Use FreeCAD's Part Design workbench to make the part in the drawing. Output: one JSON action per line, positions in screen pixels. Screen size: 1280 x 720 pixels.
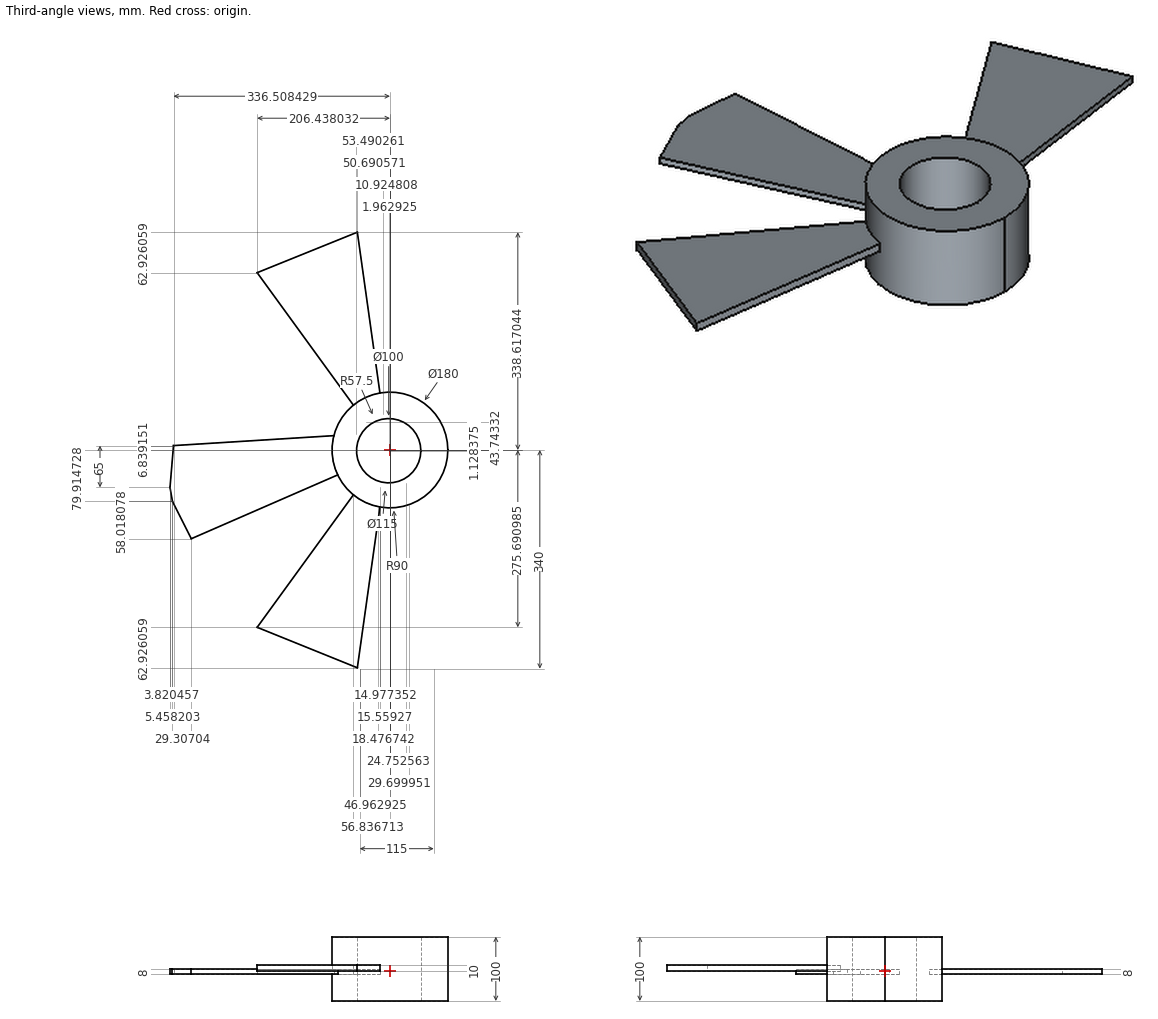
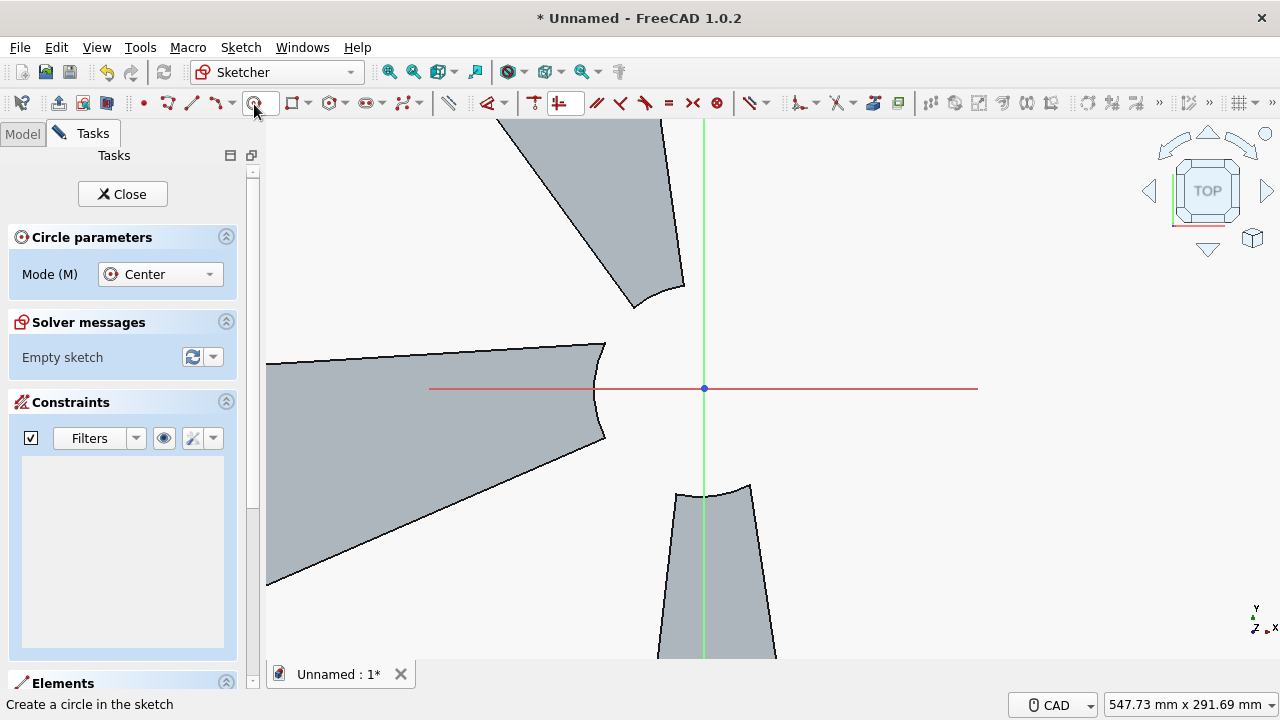
{"action": "left_click", "coordinate": [704, 389]}
{"action": "left_click", "coordinate": [822, 271]}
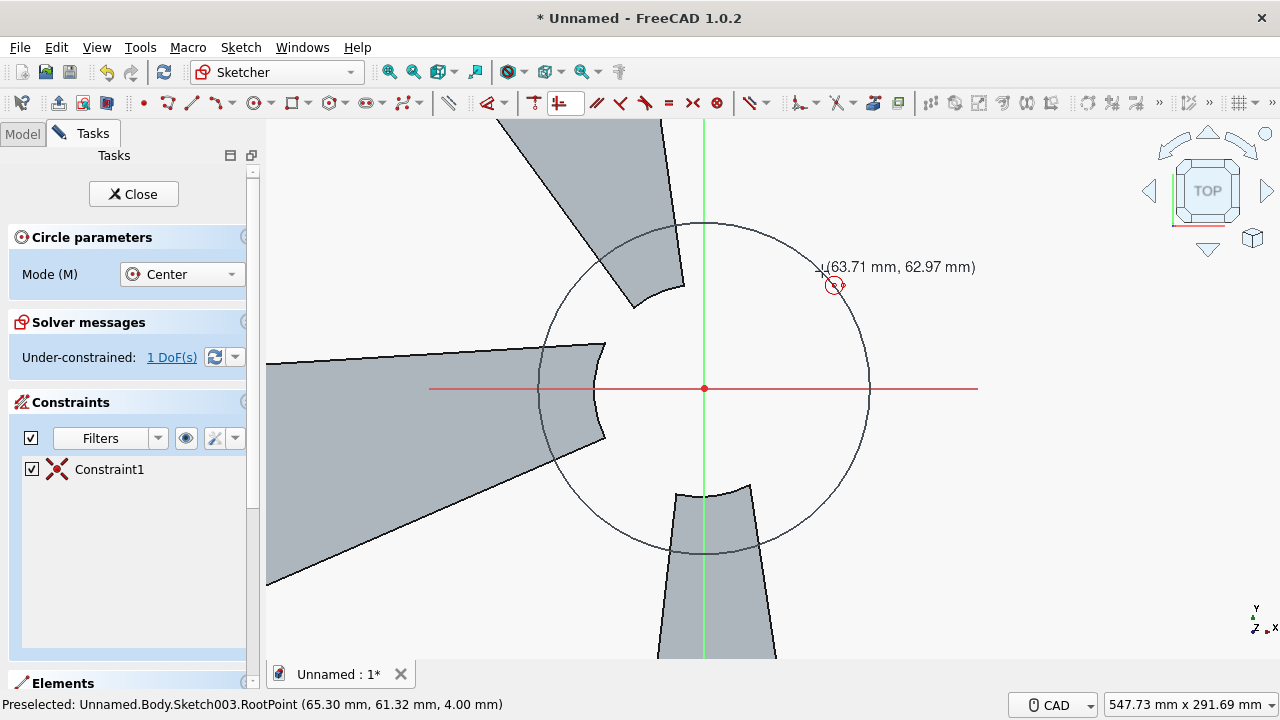
{"action": "scroll", "coordinate": [700, 391], "scroll_direction": "up", "scroll_amount": 11}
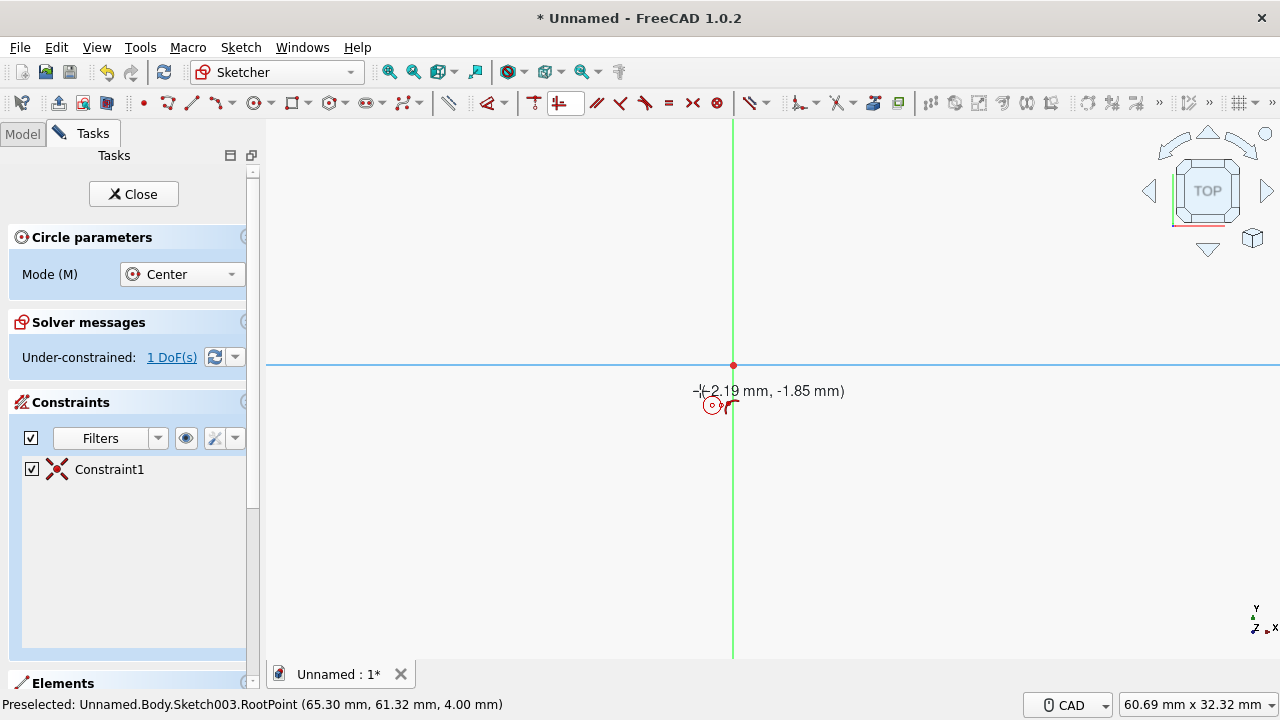
{"action": "left_click", "coordinate": [700, 384]}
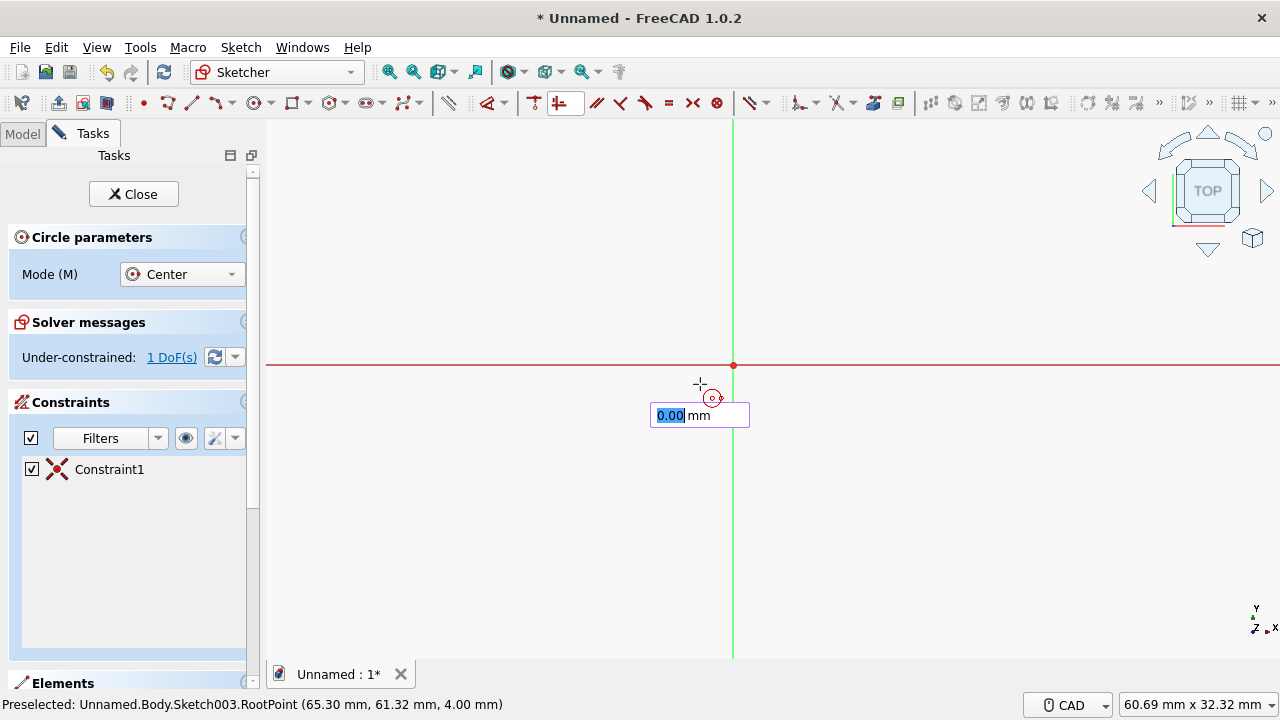
{"action": "scroll", "coordinate": [701, 392], "scroll_direction": "down", "scroll_amount": 11}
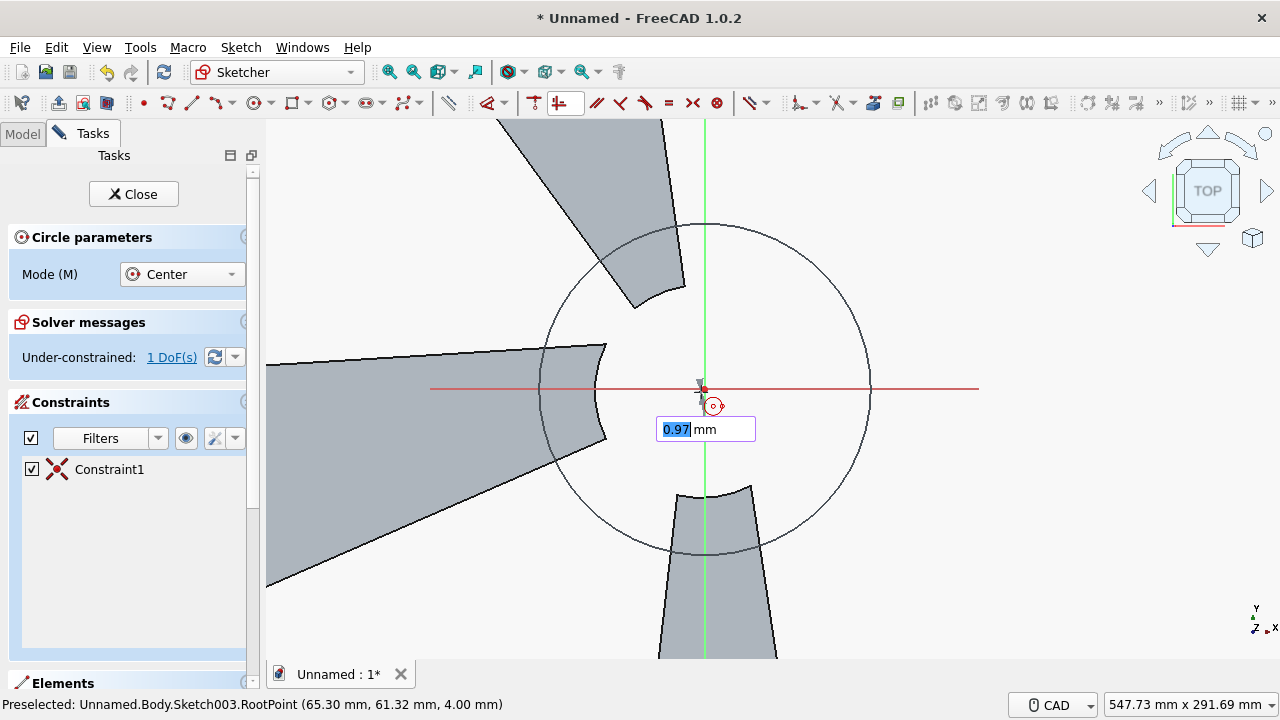
{"action": "left_click", "coordinate": [777, 316]}
{"action": "key", "text": "Escape"}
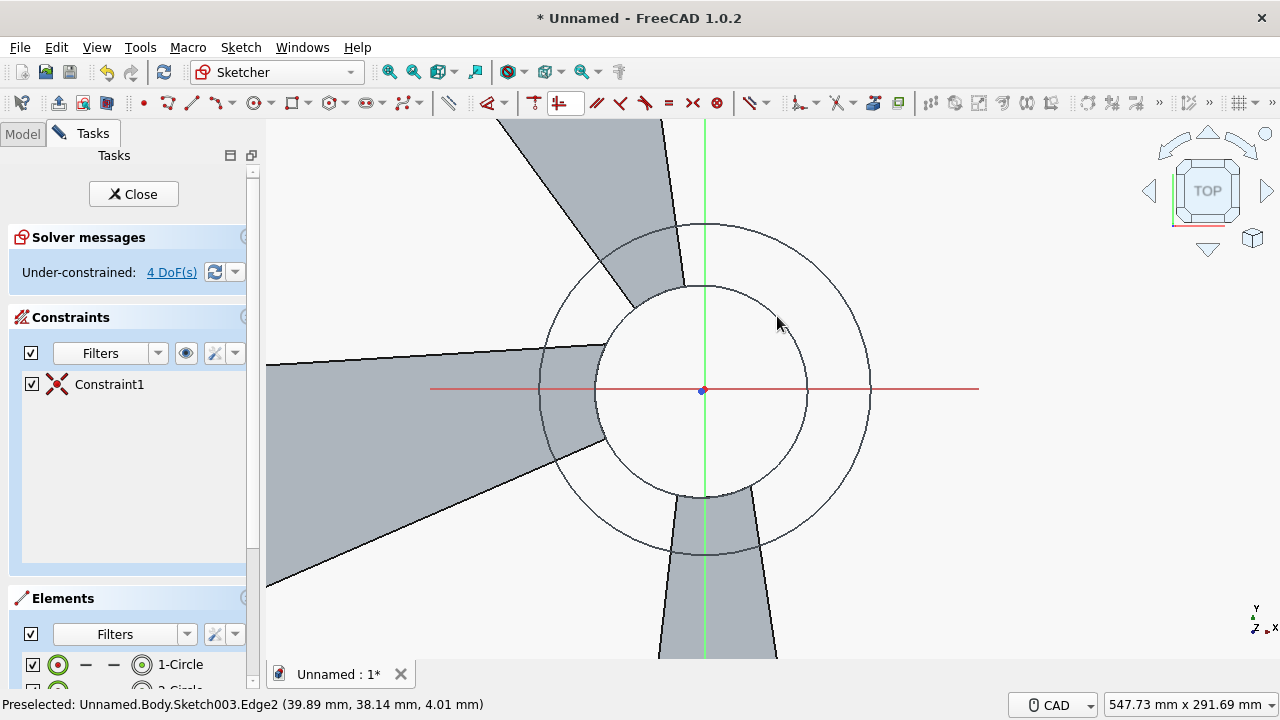
{"action": "left_click", "coordinate": [488, 104]}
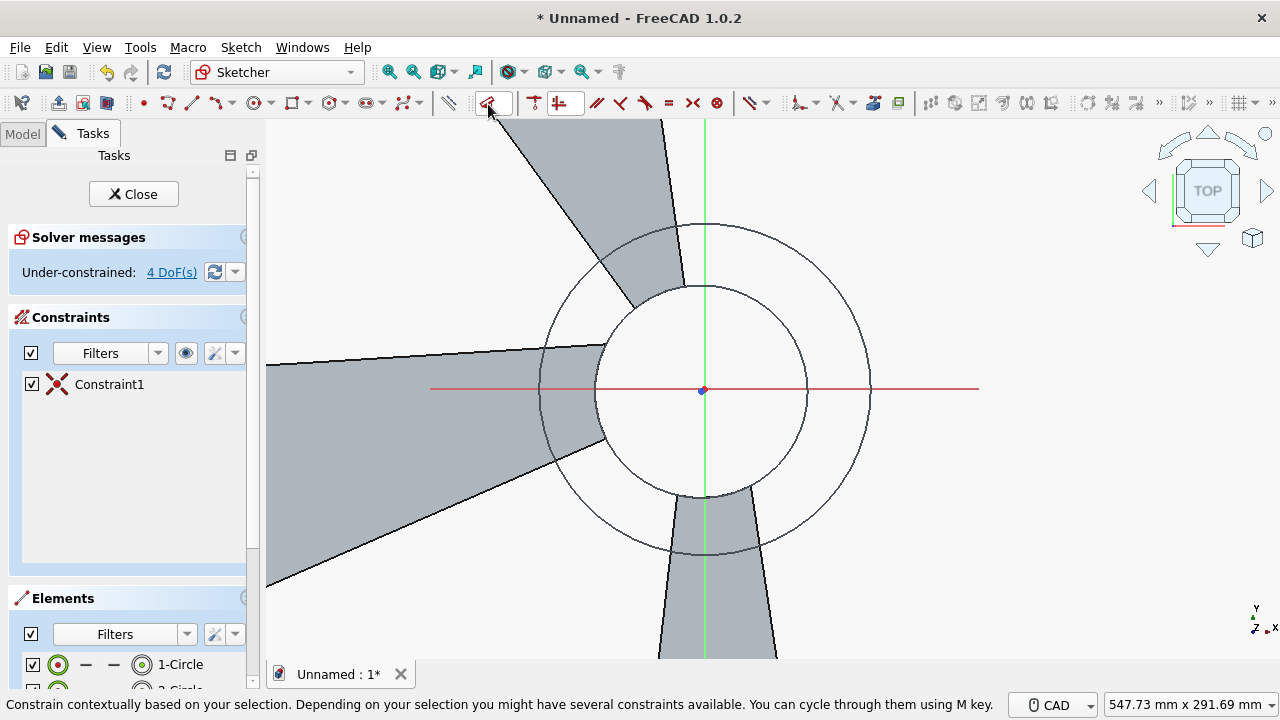
{"action": "left_click", "coordinate": [822, 272]}
{"action": "left_click", "coordinate": [845, 249]}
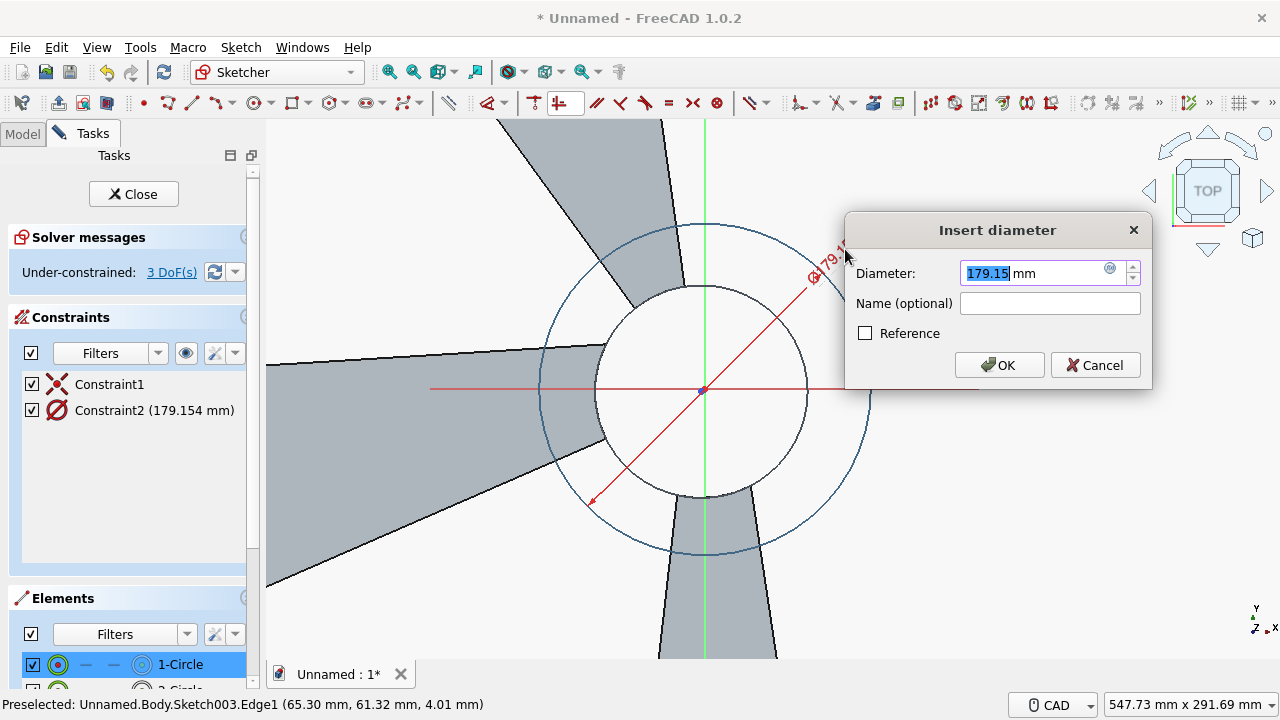
{"action": "type", "text": "180"}
{"action": "key", "text": "Return"}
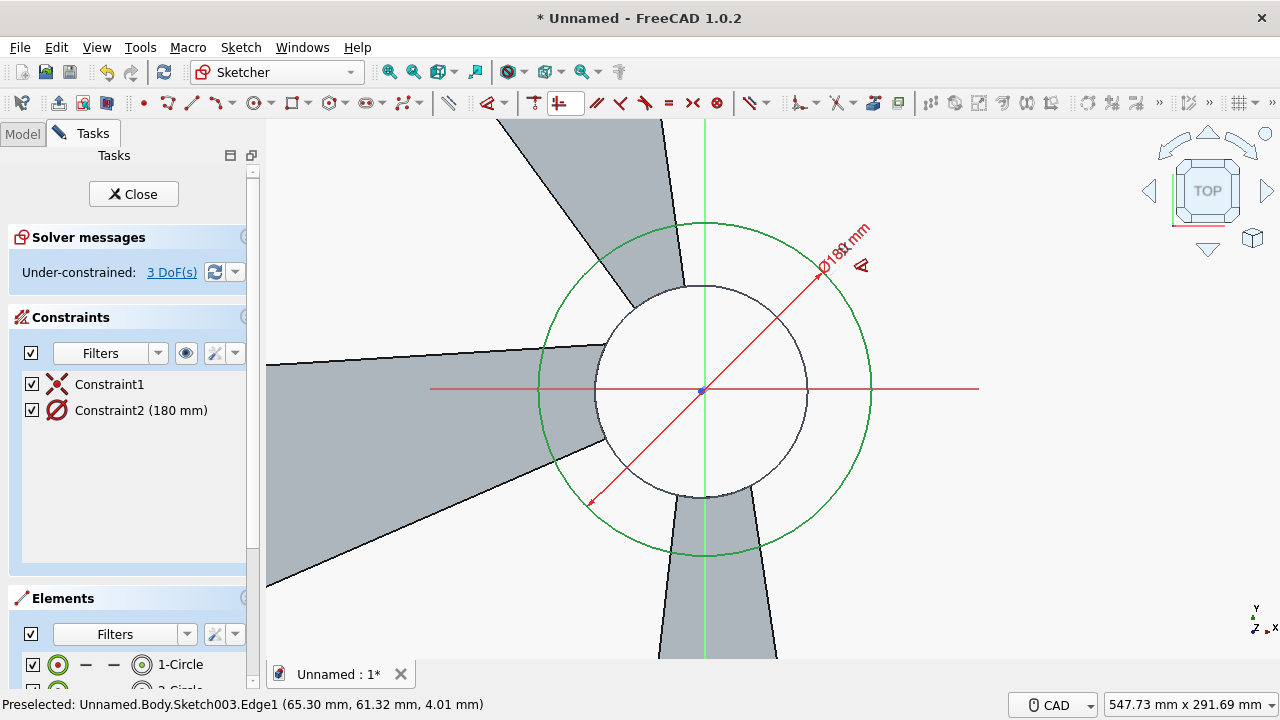
{"action": "left_click", "coordinate": [776, 316]}
{"action": "left_click", "coordinate": [798, 293]}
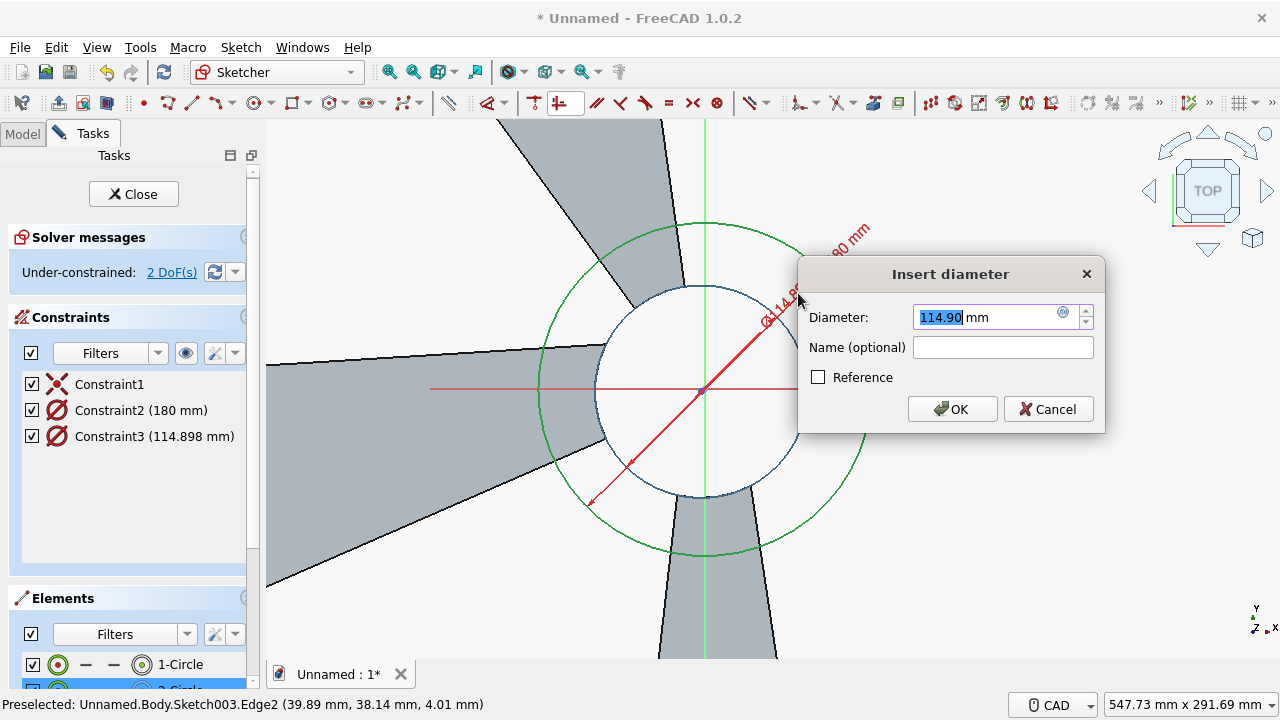
{"action": "type", "text": "115"}
{"action": "key", "text": "Return"}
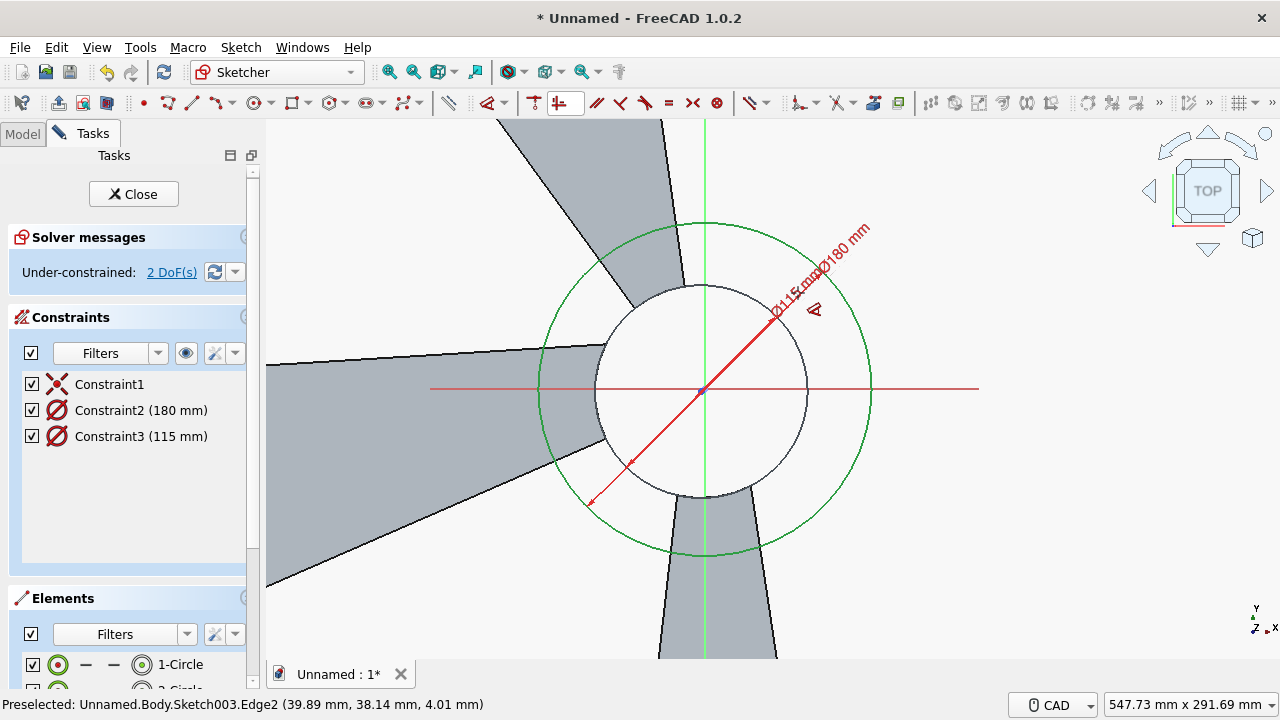
{"action": "scroll", "coordinate": [701, 392], "scroll_direction": "up", "scroll_amount": 12}